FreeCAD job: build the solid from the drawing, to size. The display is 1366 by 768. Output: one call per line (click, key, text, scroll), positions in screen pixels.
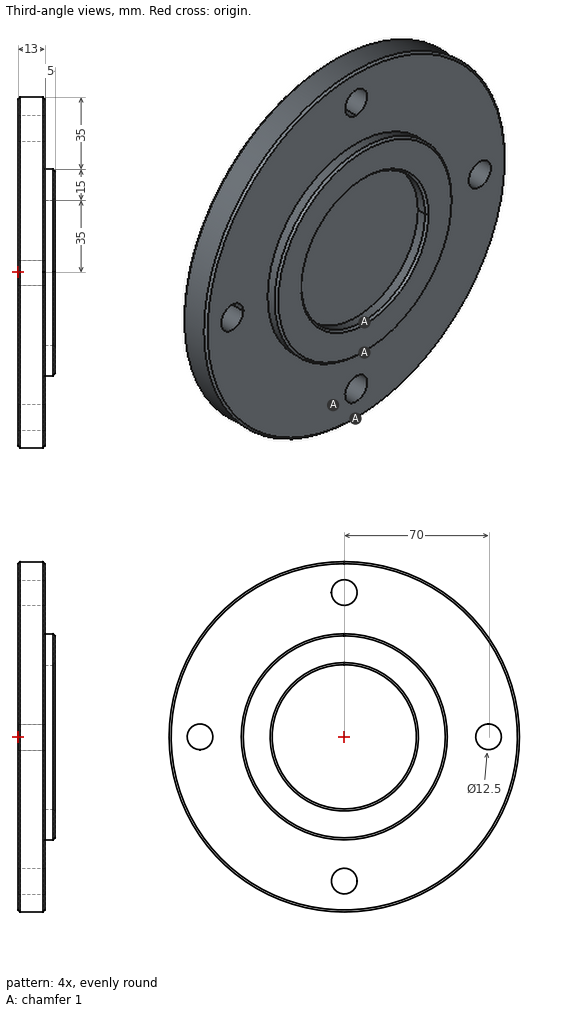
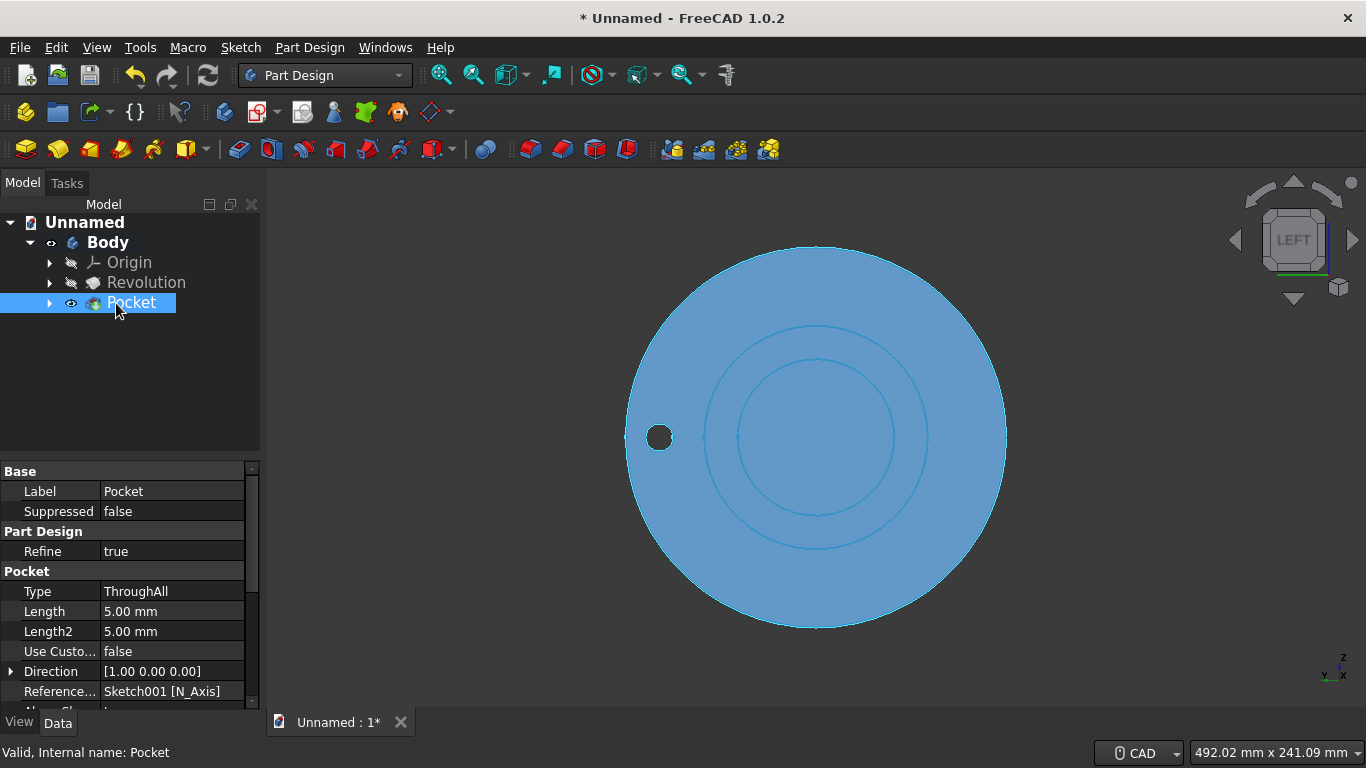
click(736, 150)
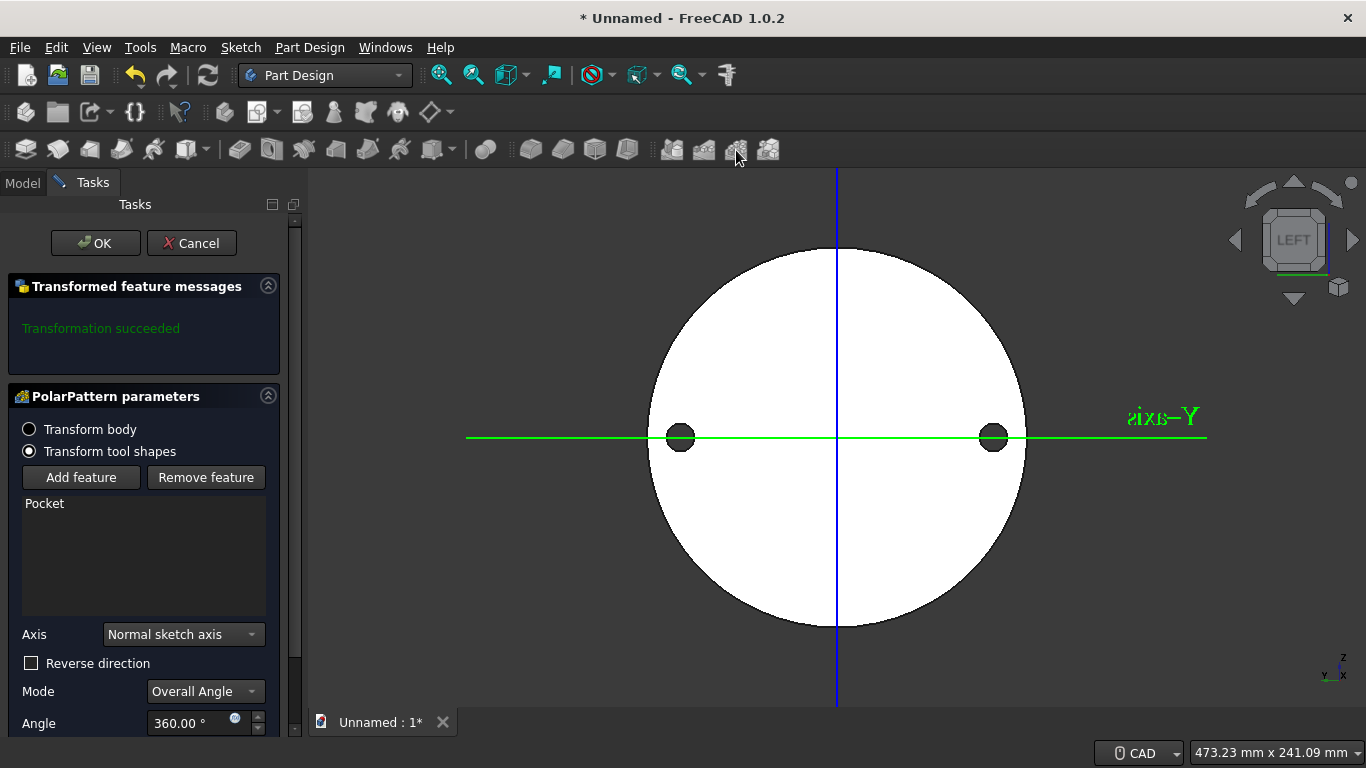
click(184, 634)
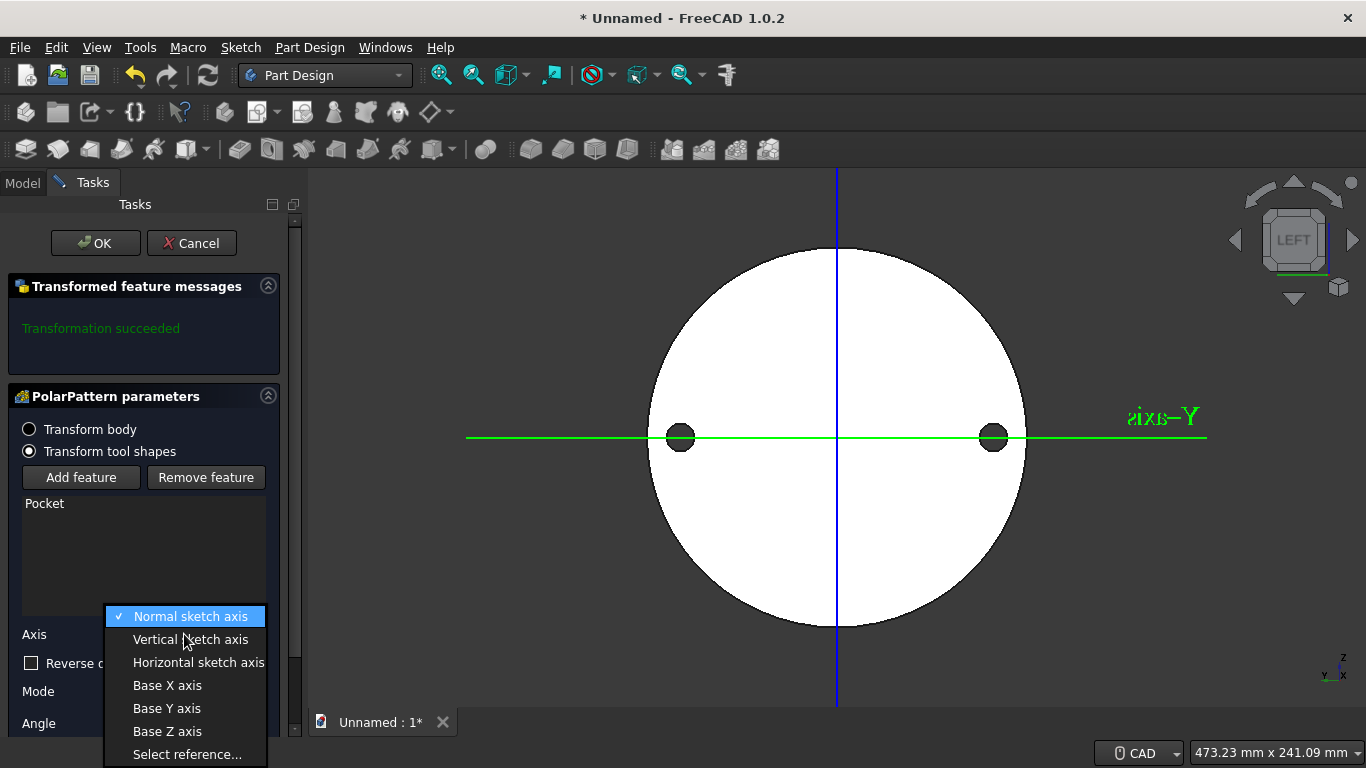
click(184, 686)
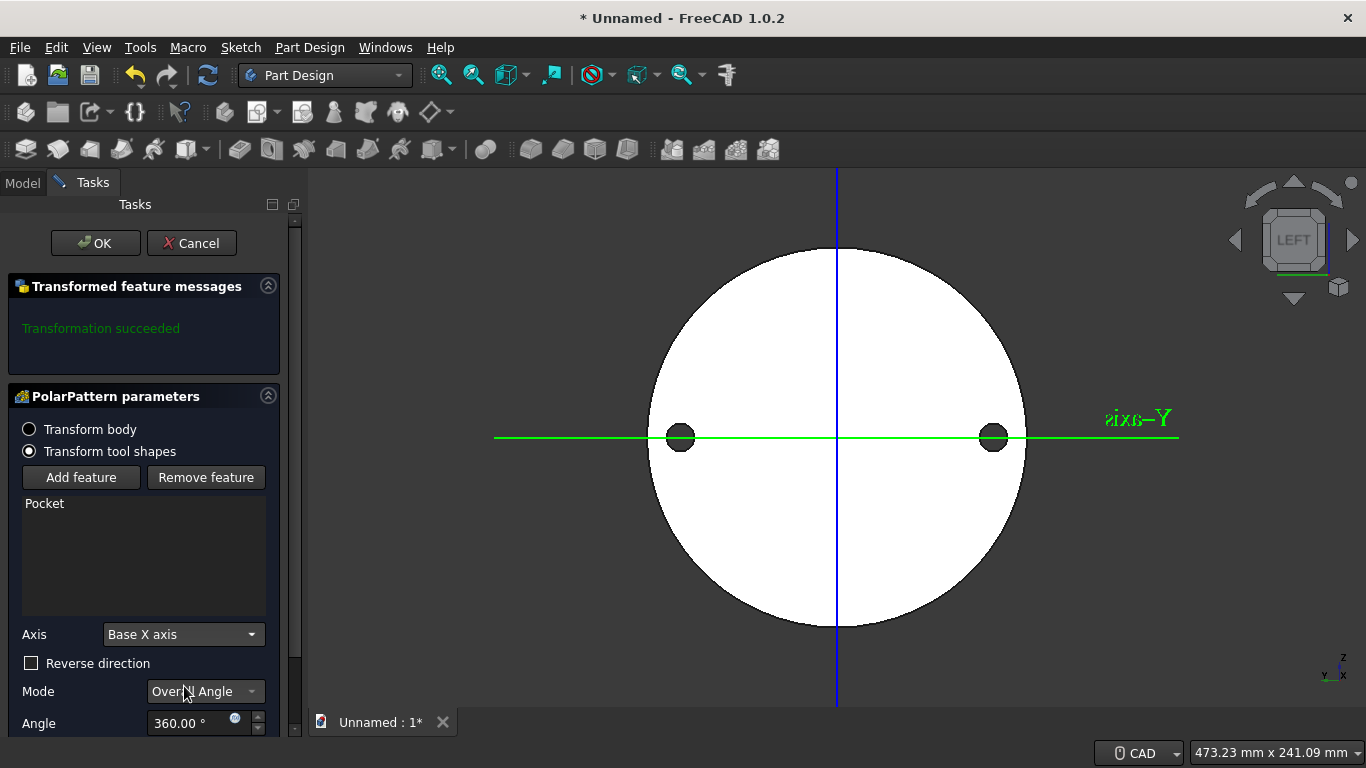
scroll(295, 475, down, 2)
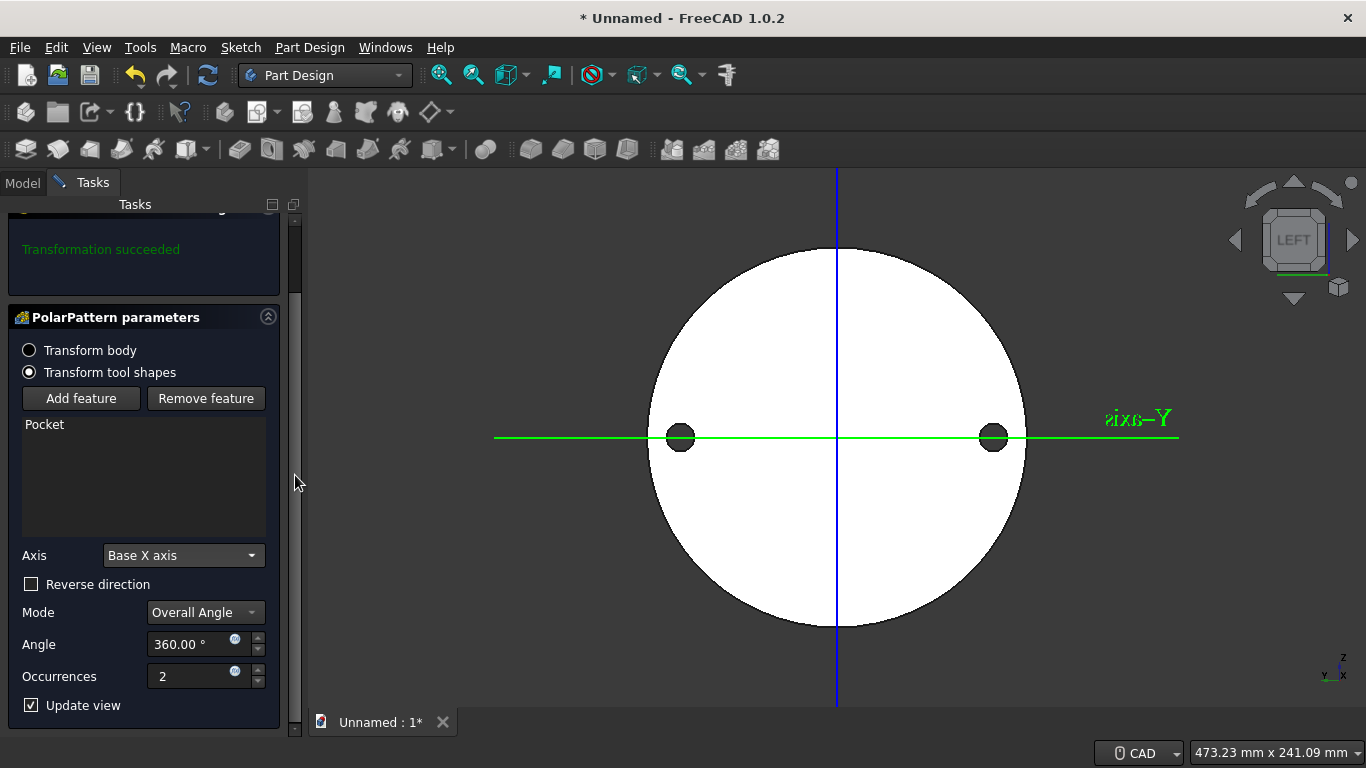
triple_click(198, 676)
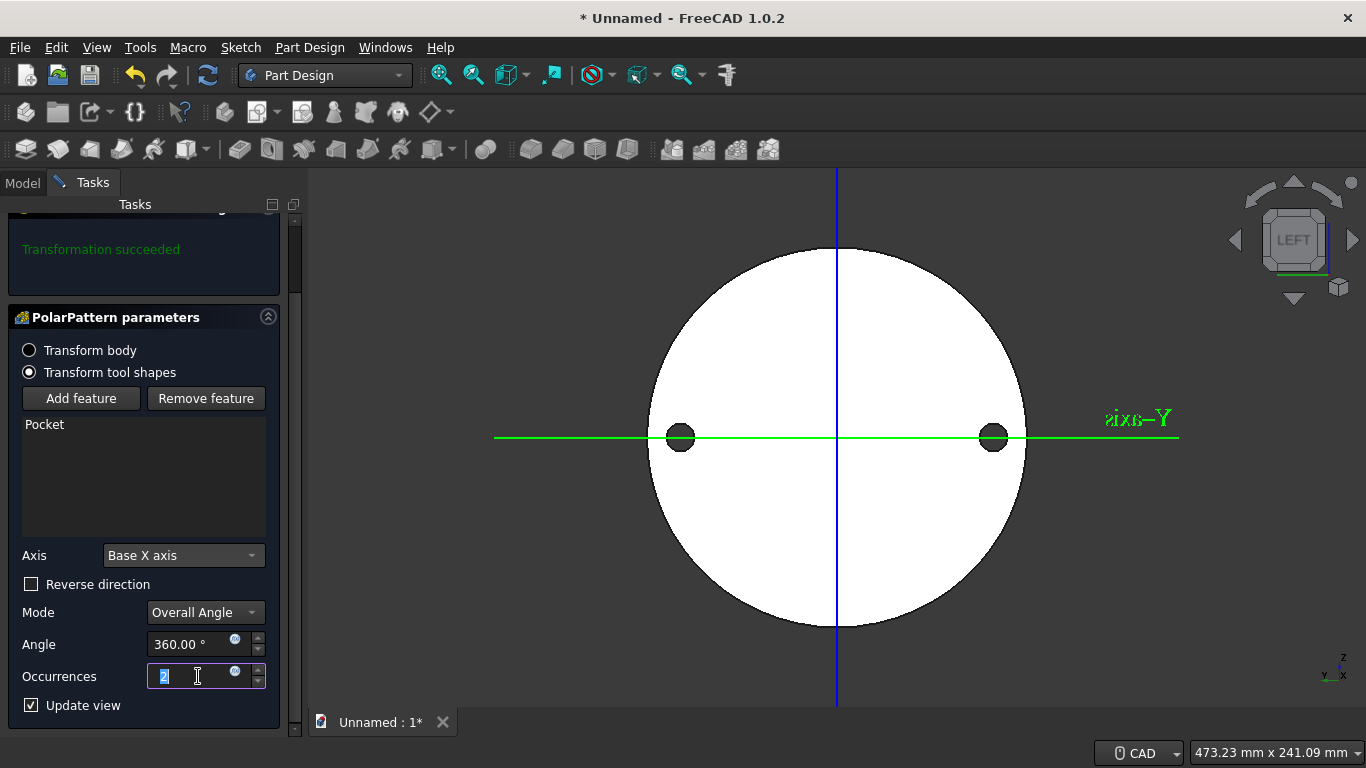
text(4)
key(Tab)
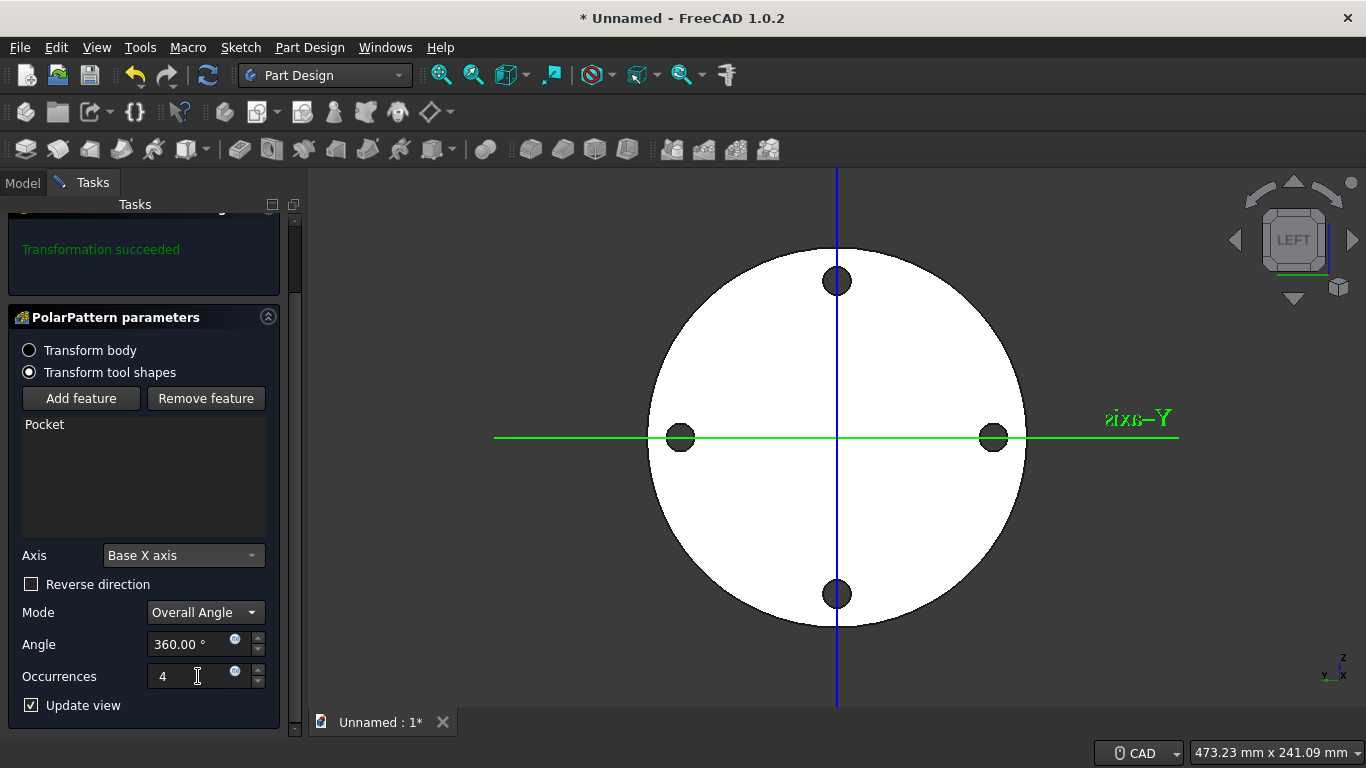
scroll(295, 475, up, 3)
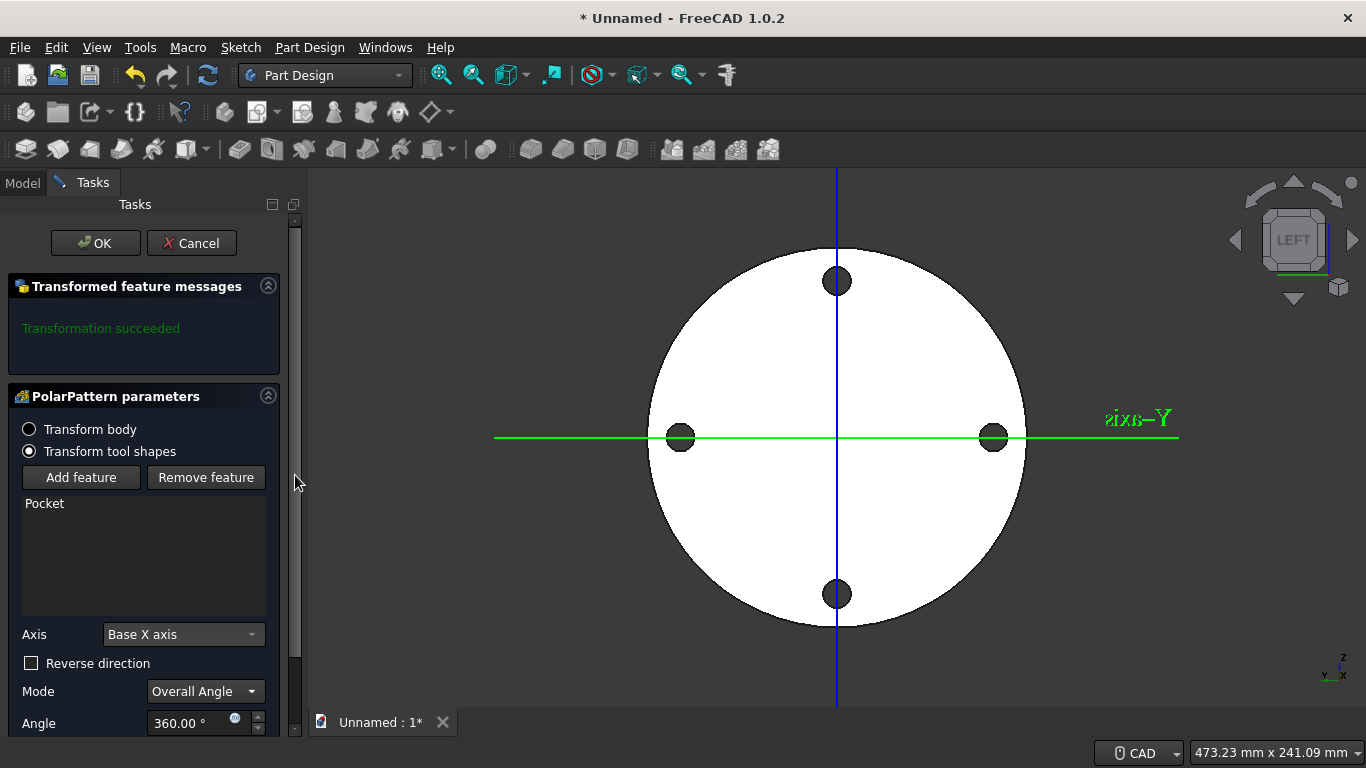
click(96, 243)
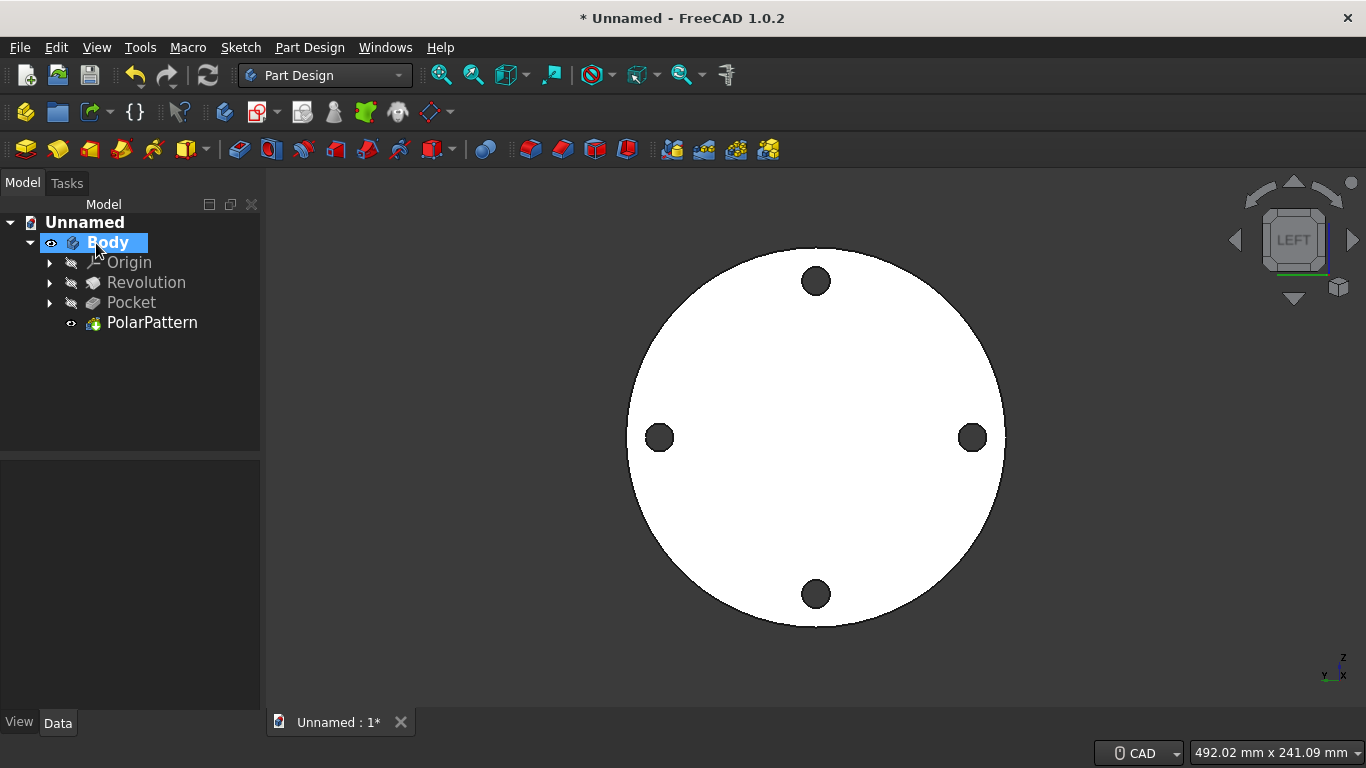
click(1006, 436)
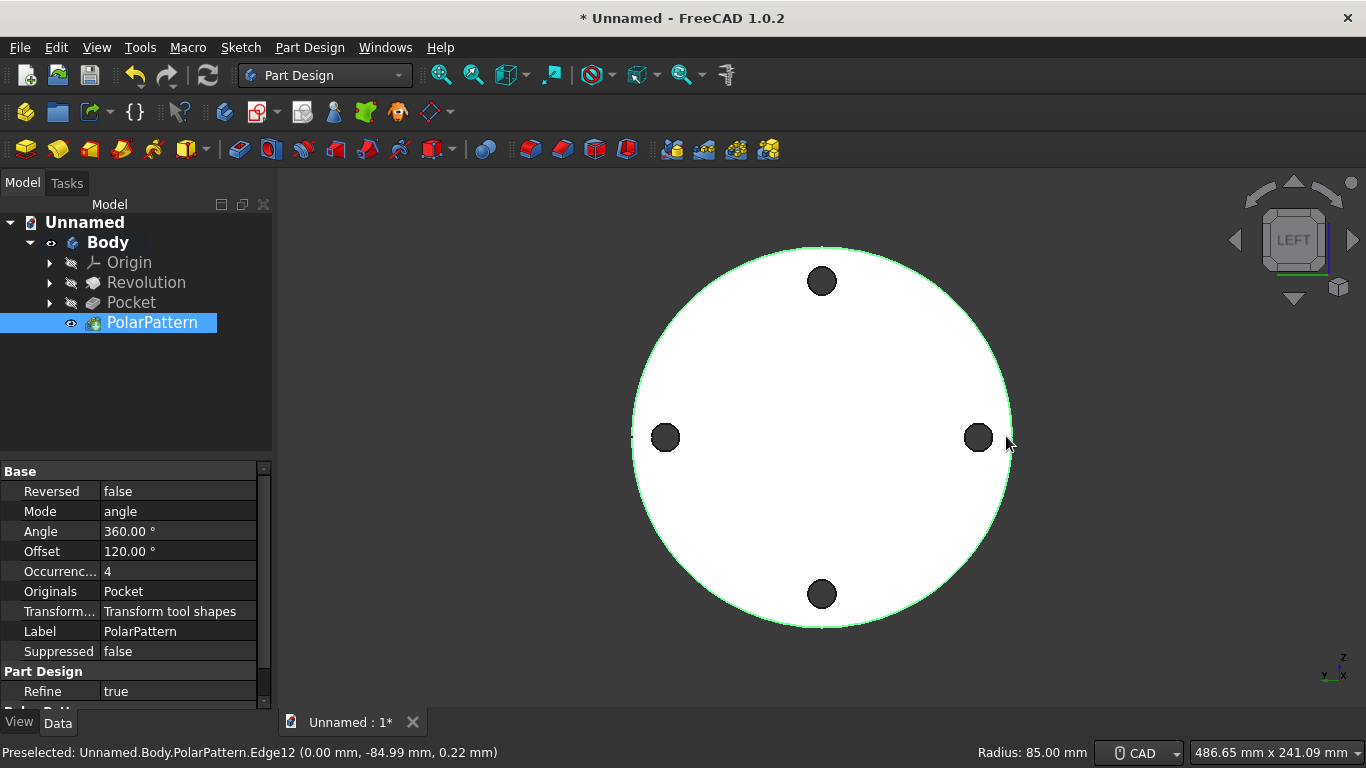
key(0)